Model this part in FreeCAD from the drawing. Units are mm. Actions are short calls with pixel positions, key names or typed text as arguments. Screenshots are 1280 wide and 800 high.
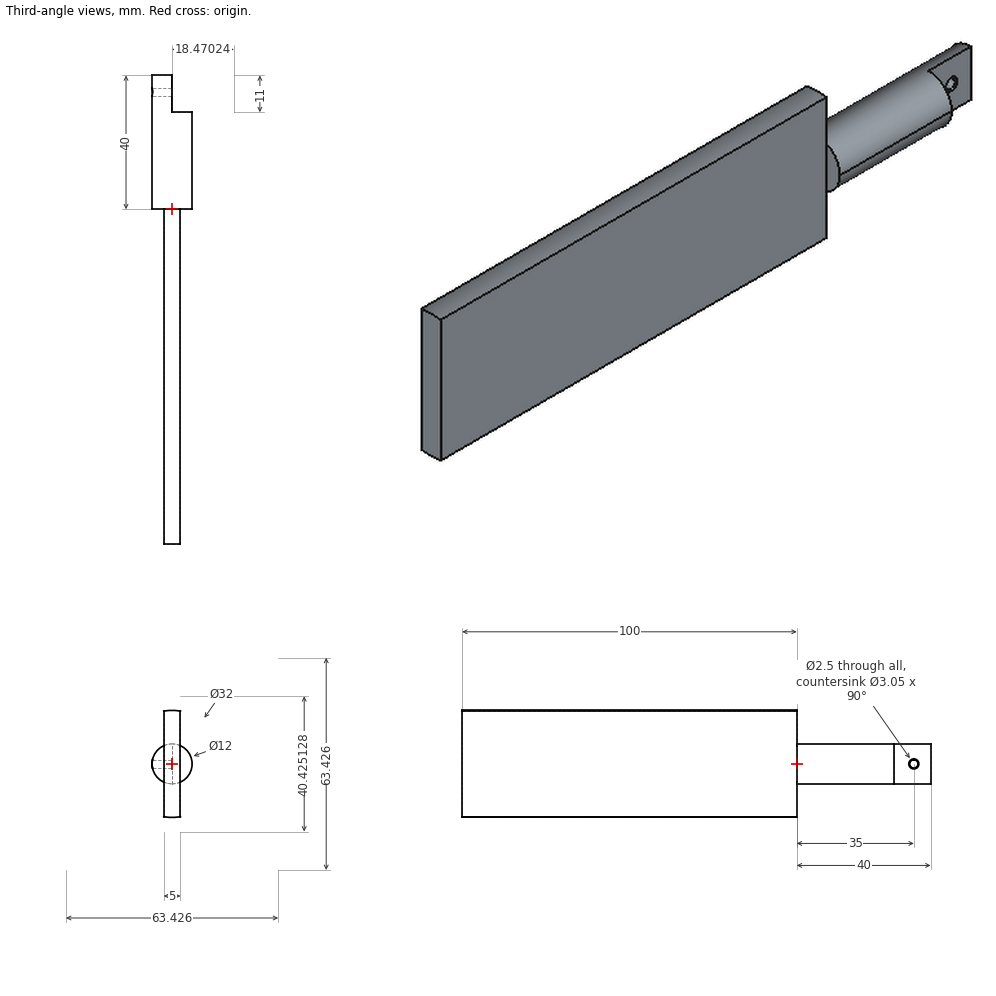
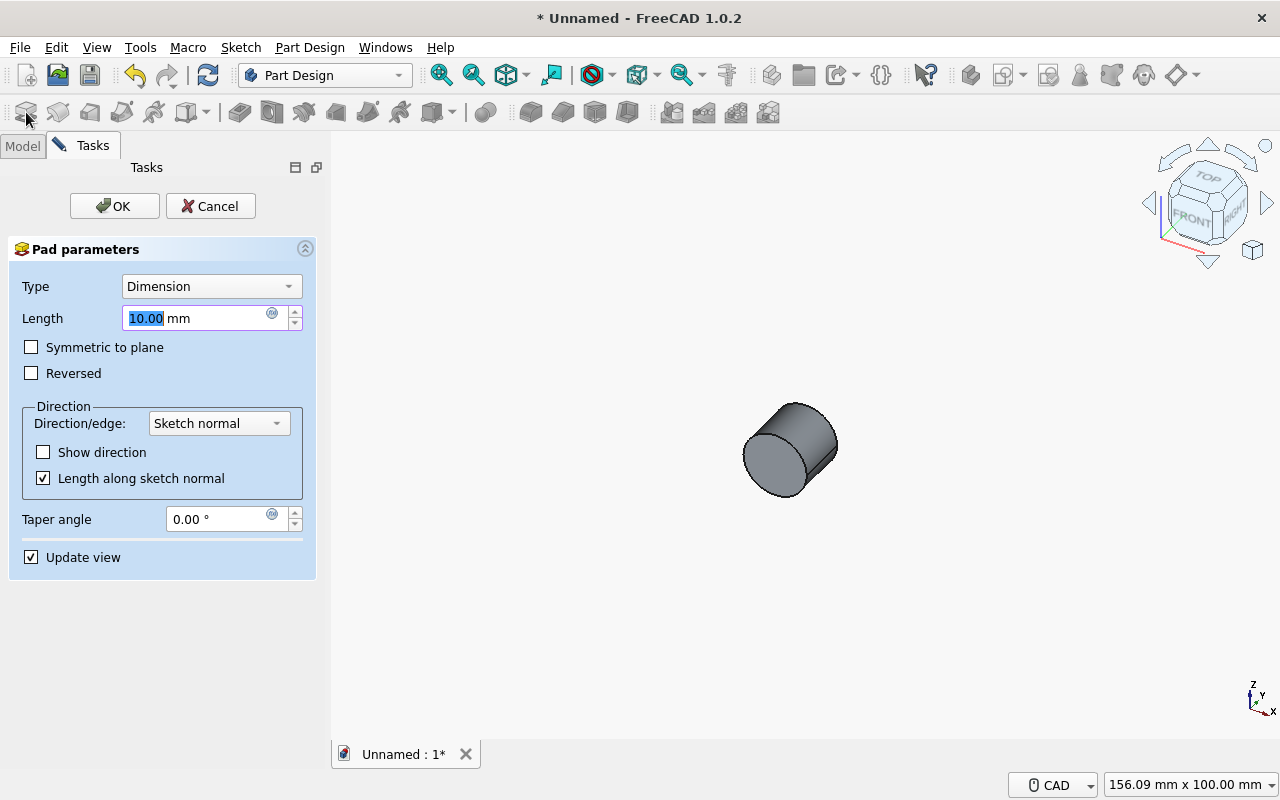
text(40)
key(Tab)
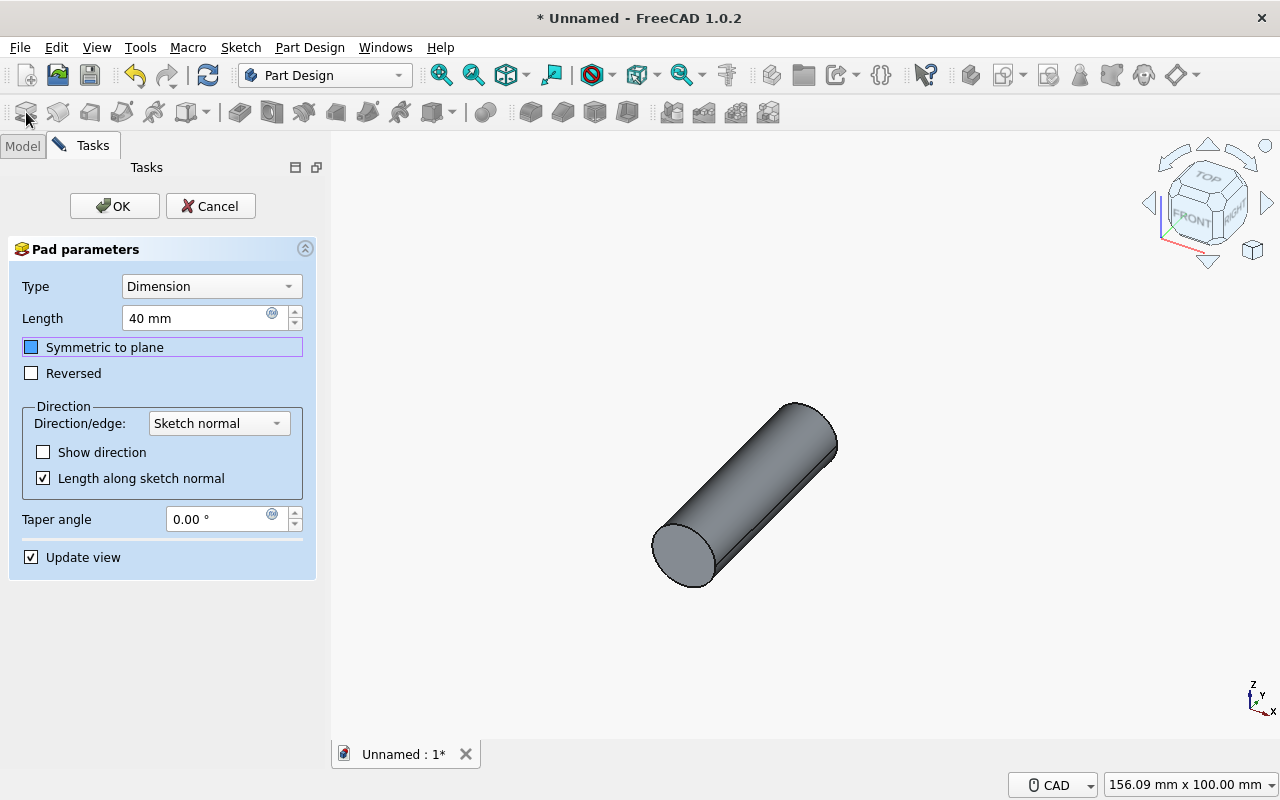
click(30, 373)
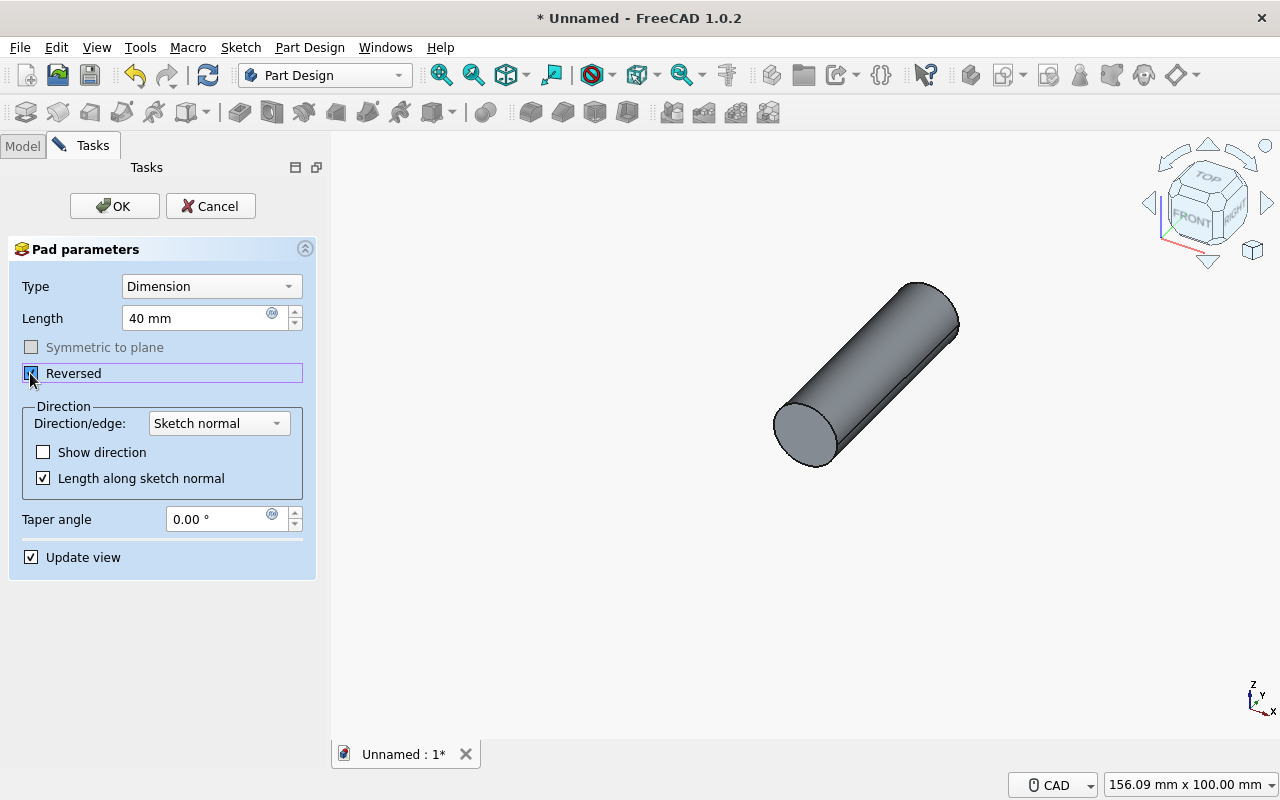
click(115, 206)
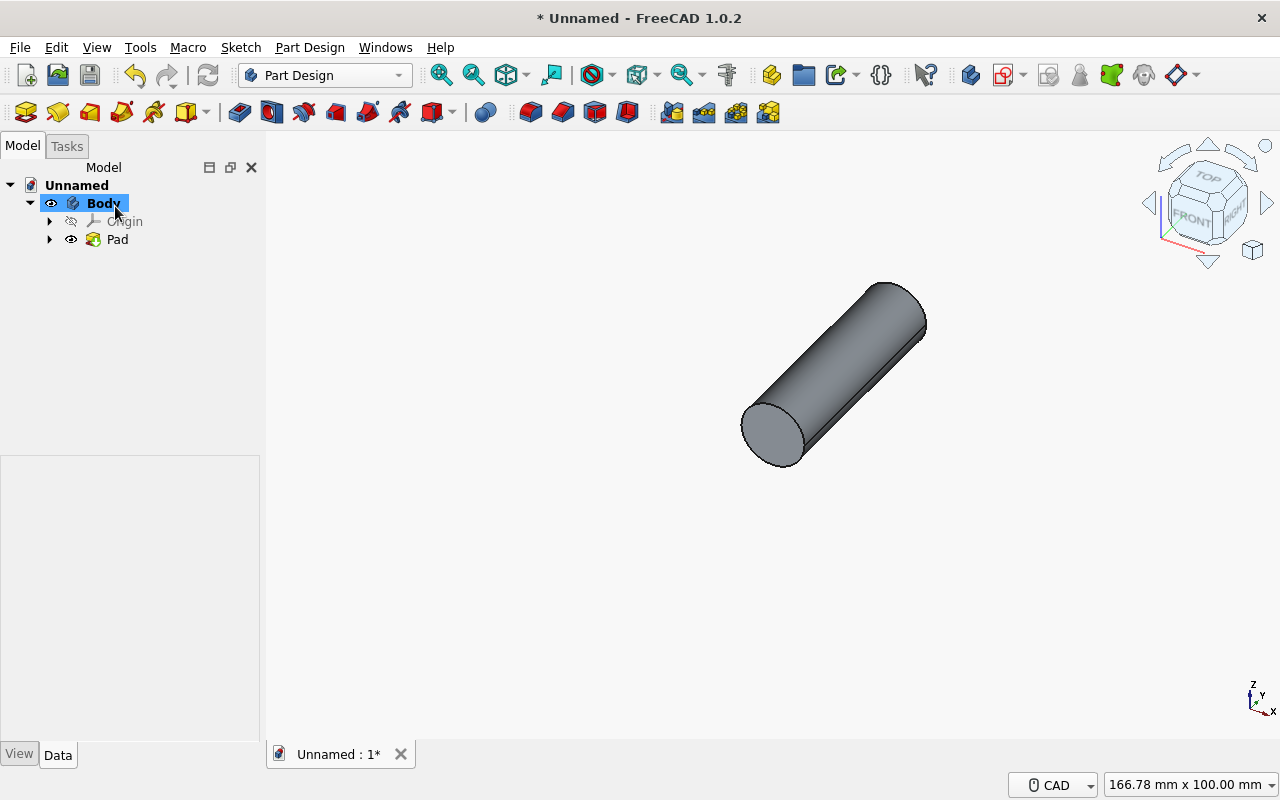
click(442, 76)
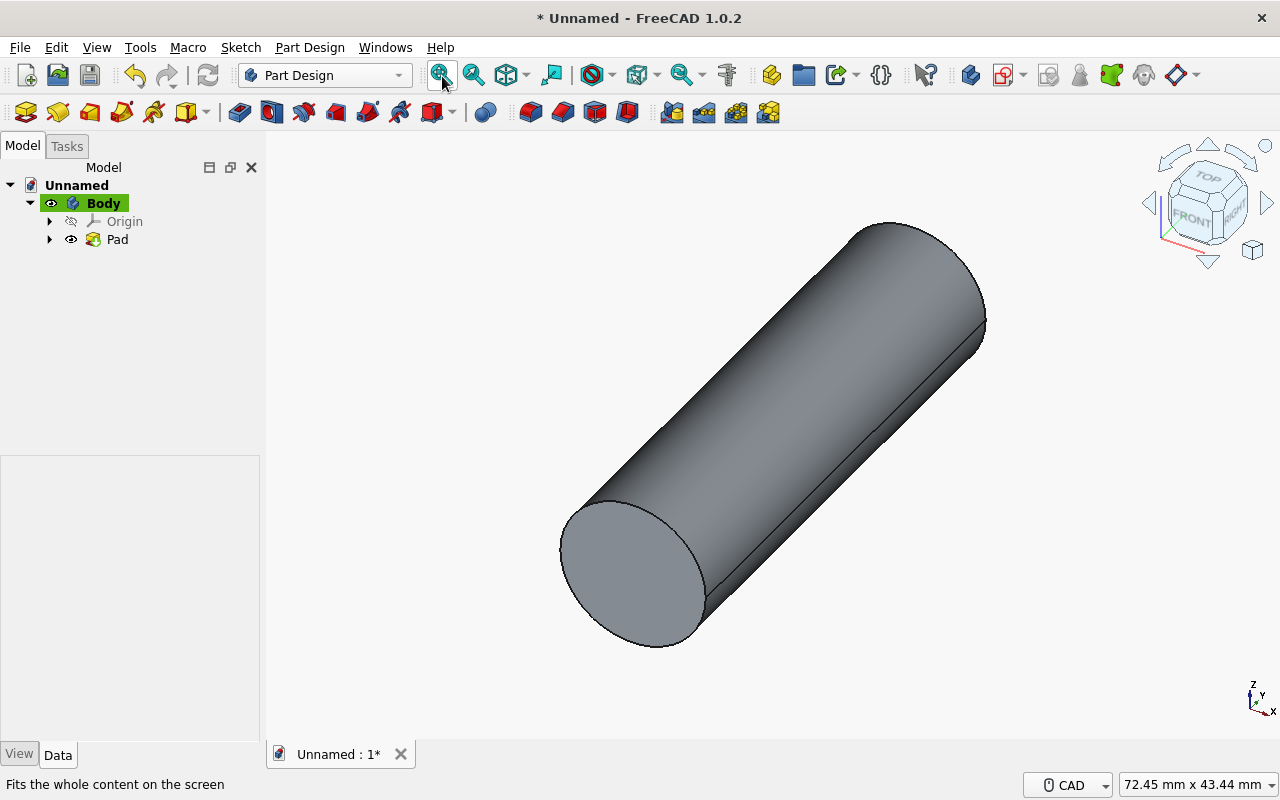
click(1004, 76)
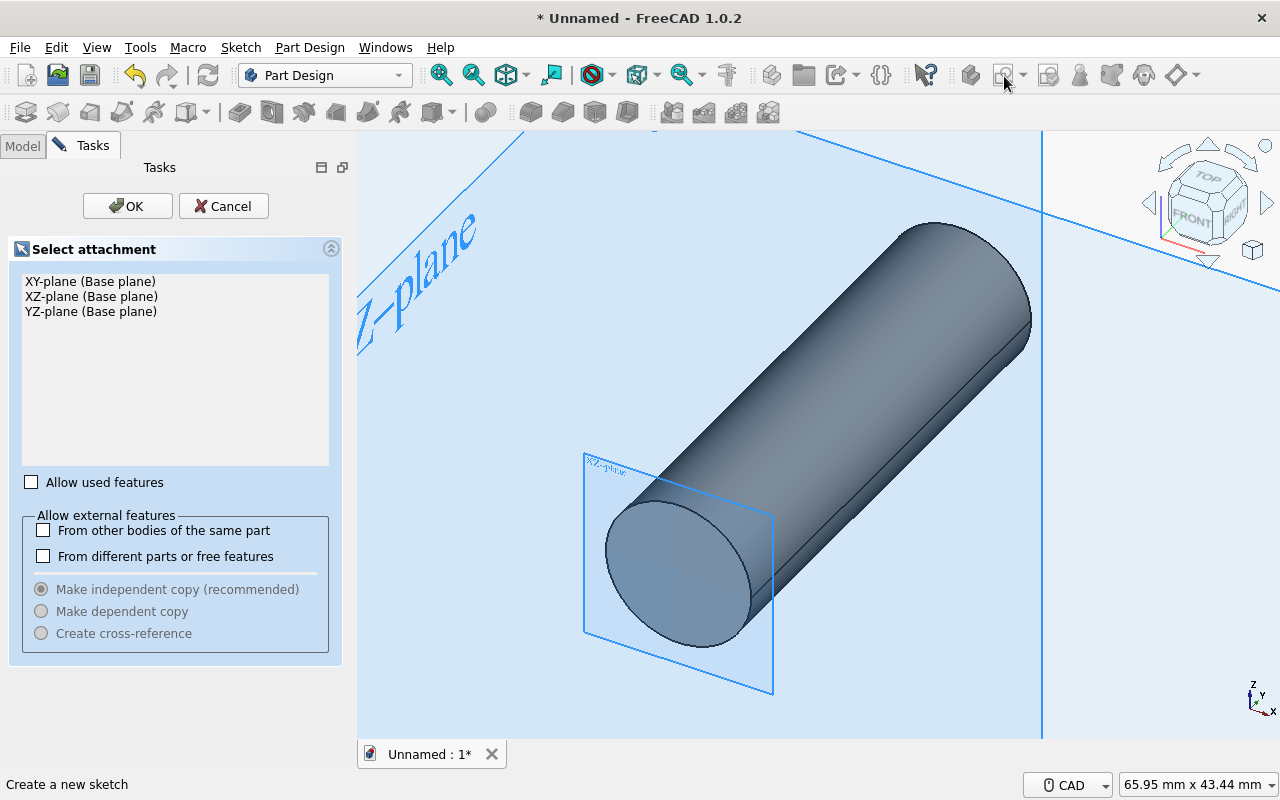
click(82, 282)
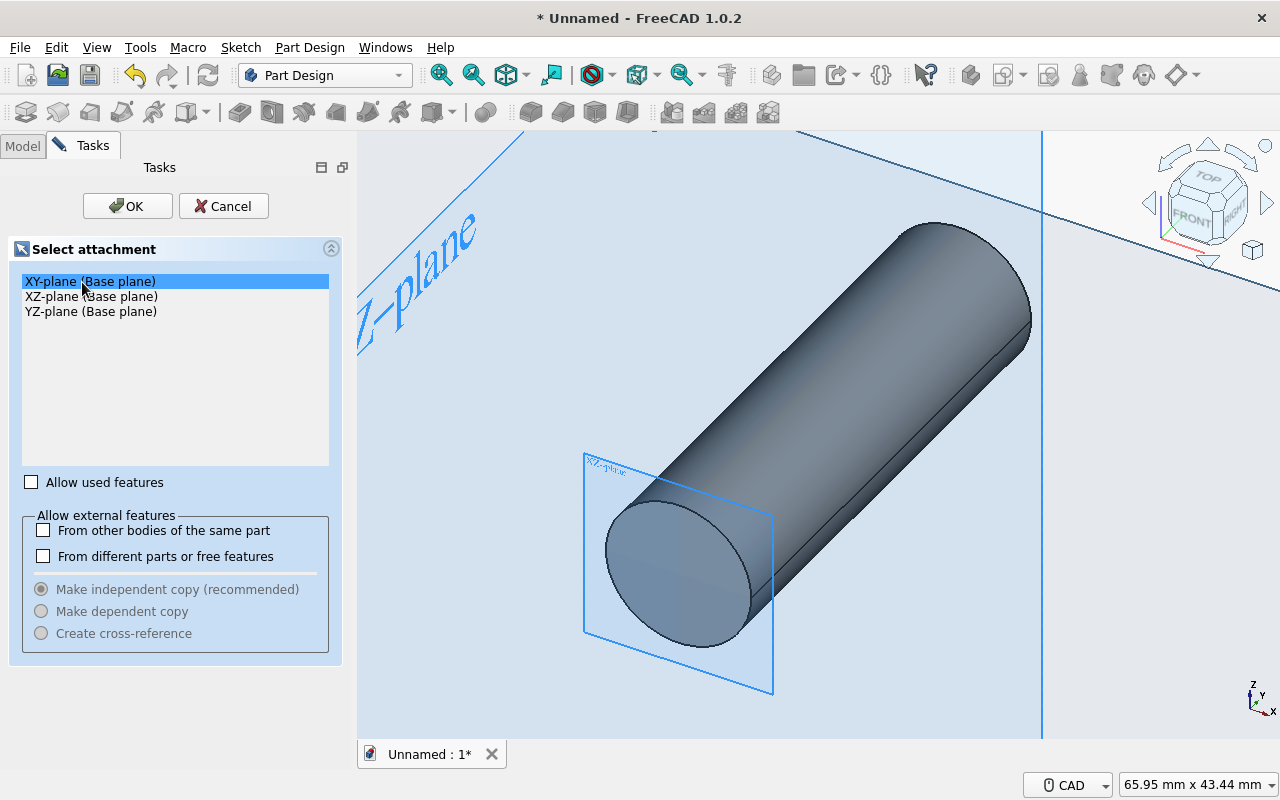
click(128, 206)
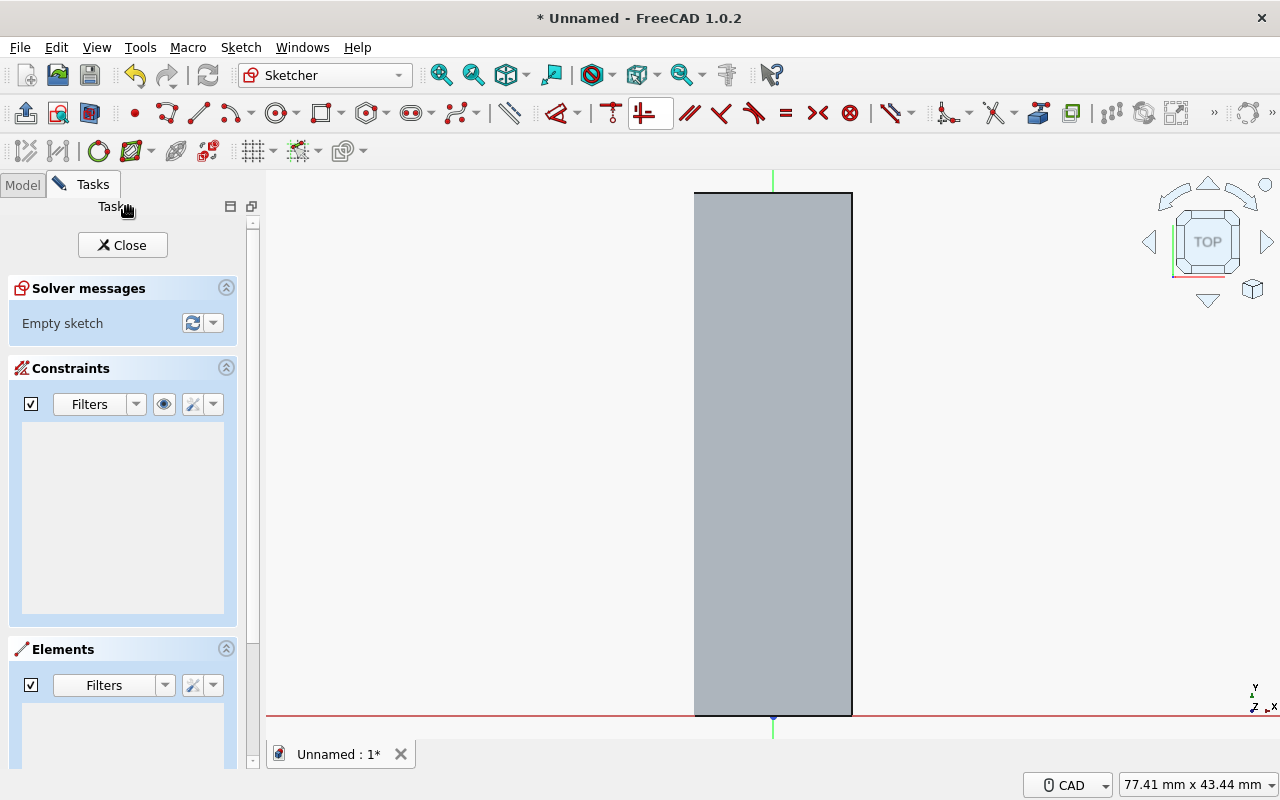
click(90, 114)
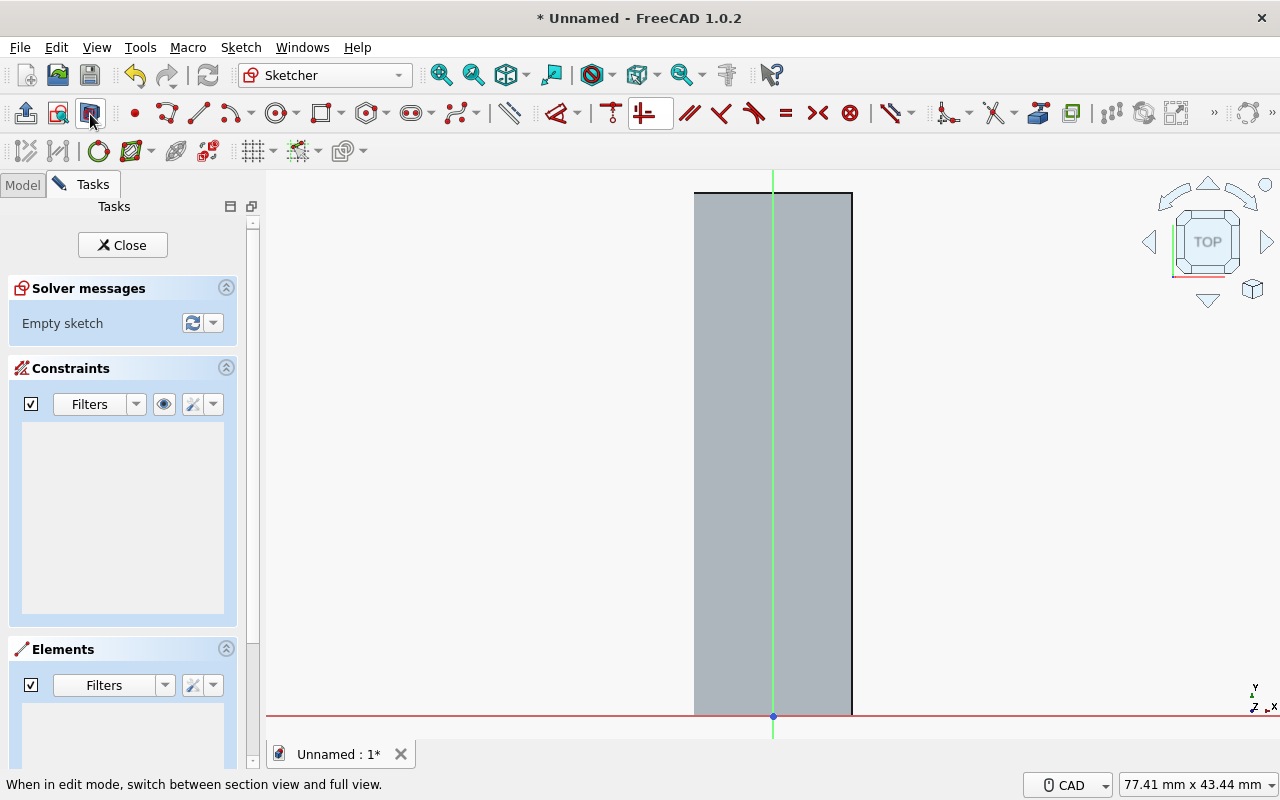
scroll(319, 454, down, 2)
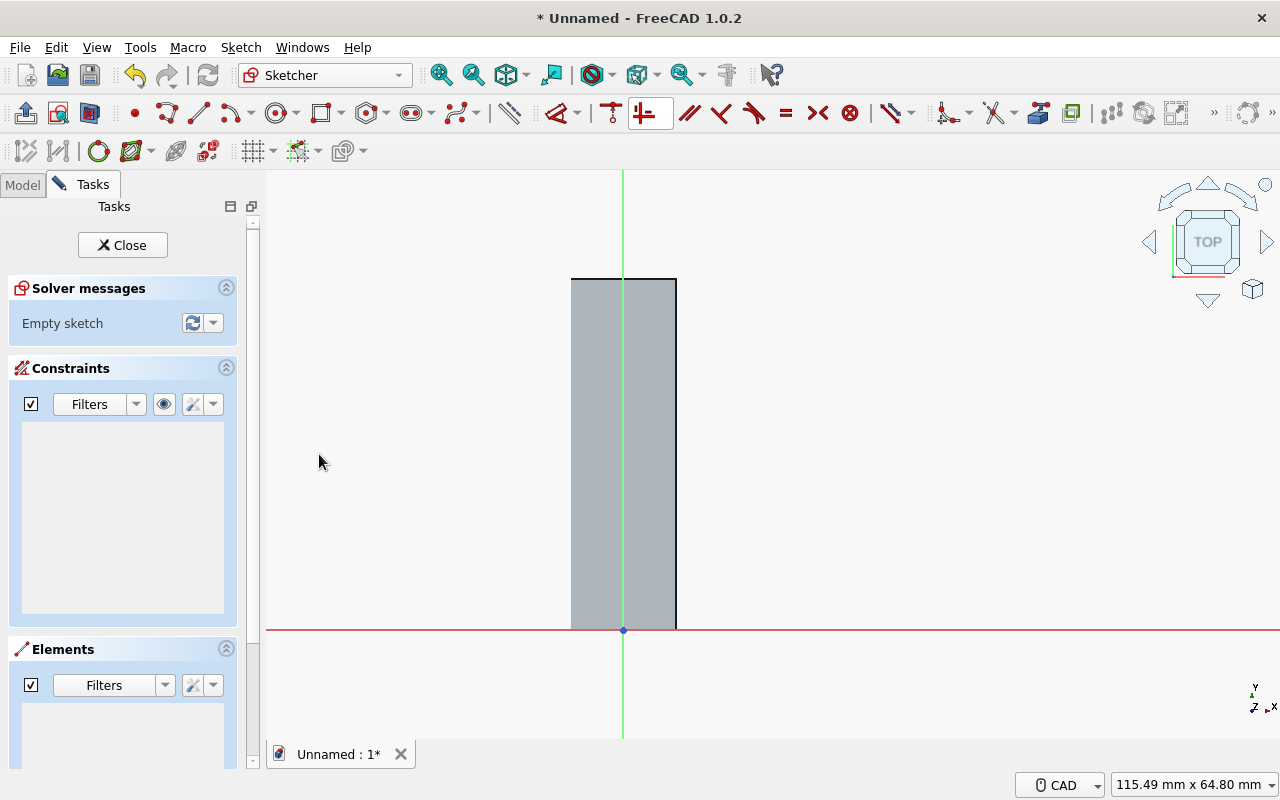
click(322, 114)